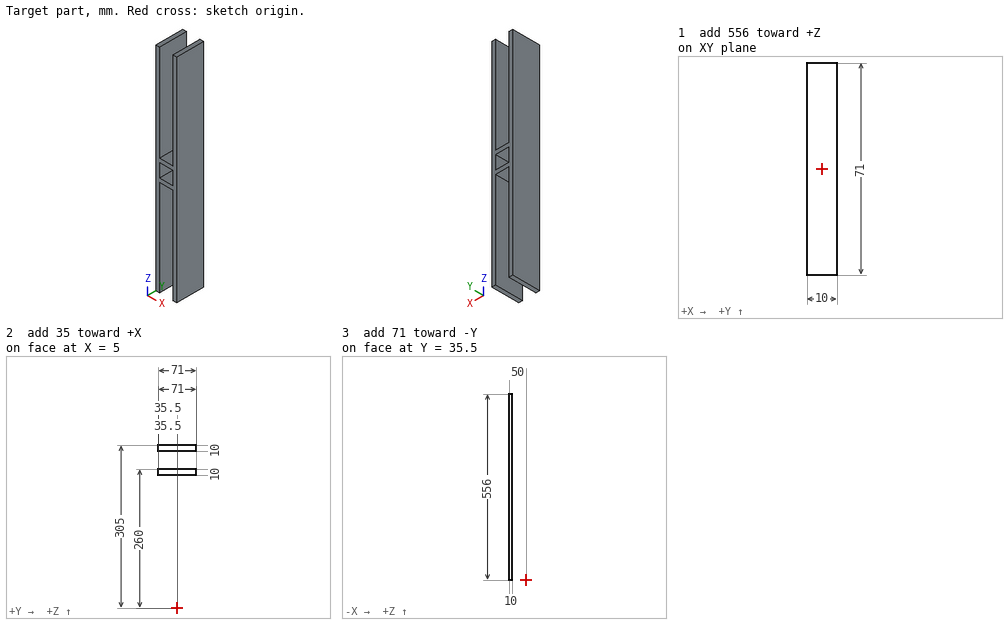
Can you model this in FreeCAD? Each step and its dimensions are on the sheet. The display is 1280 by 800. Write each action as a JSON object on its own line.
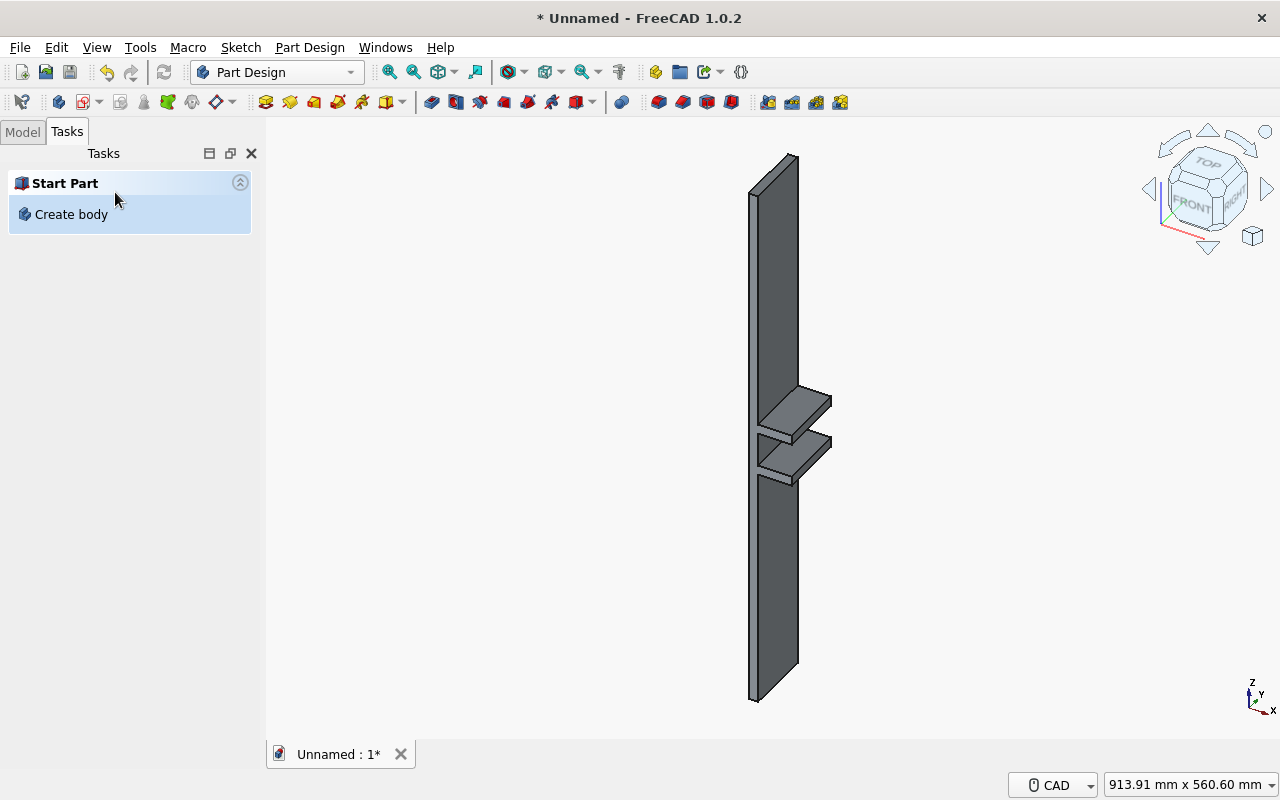
{"action": "key", "text": "4"}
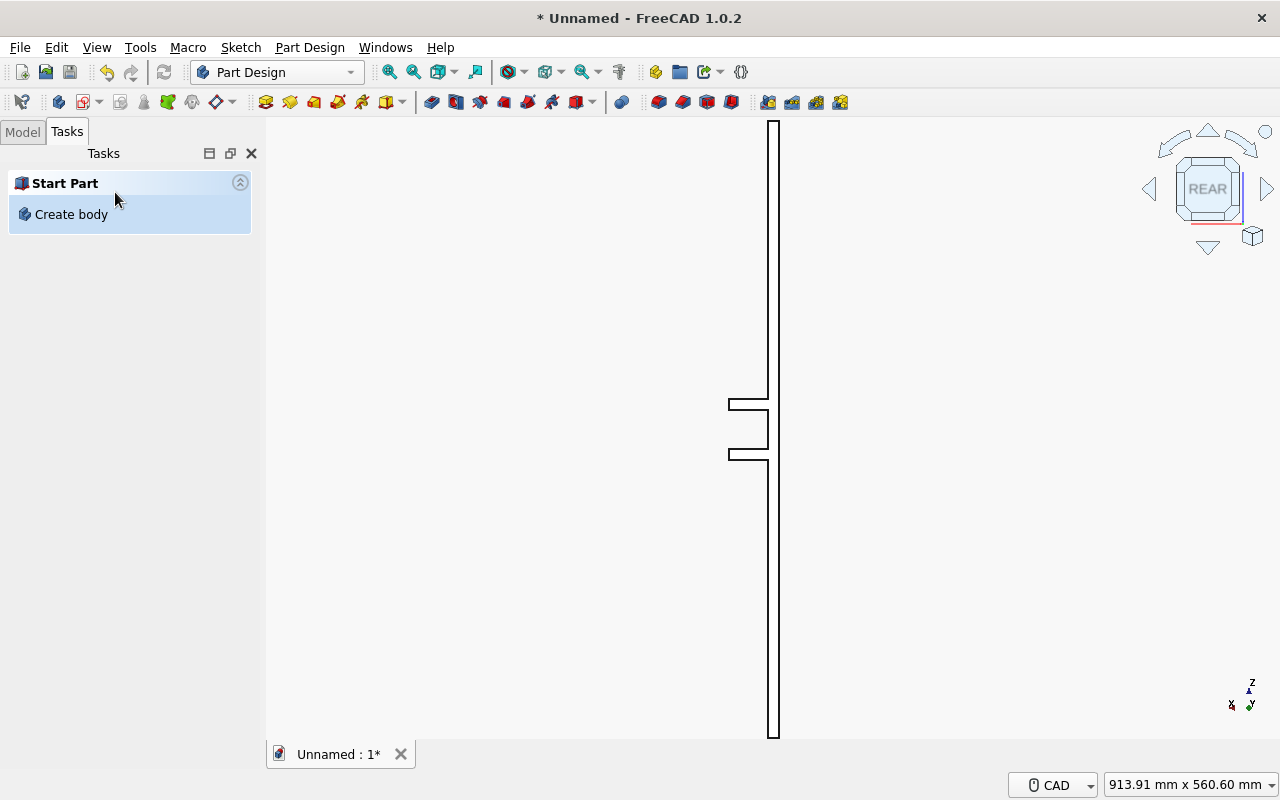
{"action": "scroll", "coordinate": [776, 164], "scroll_direction": "up", "scroll_amount": 7}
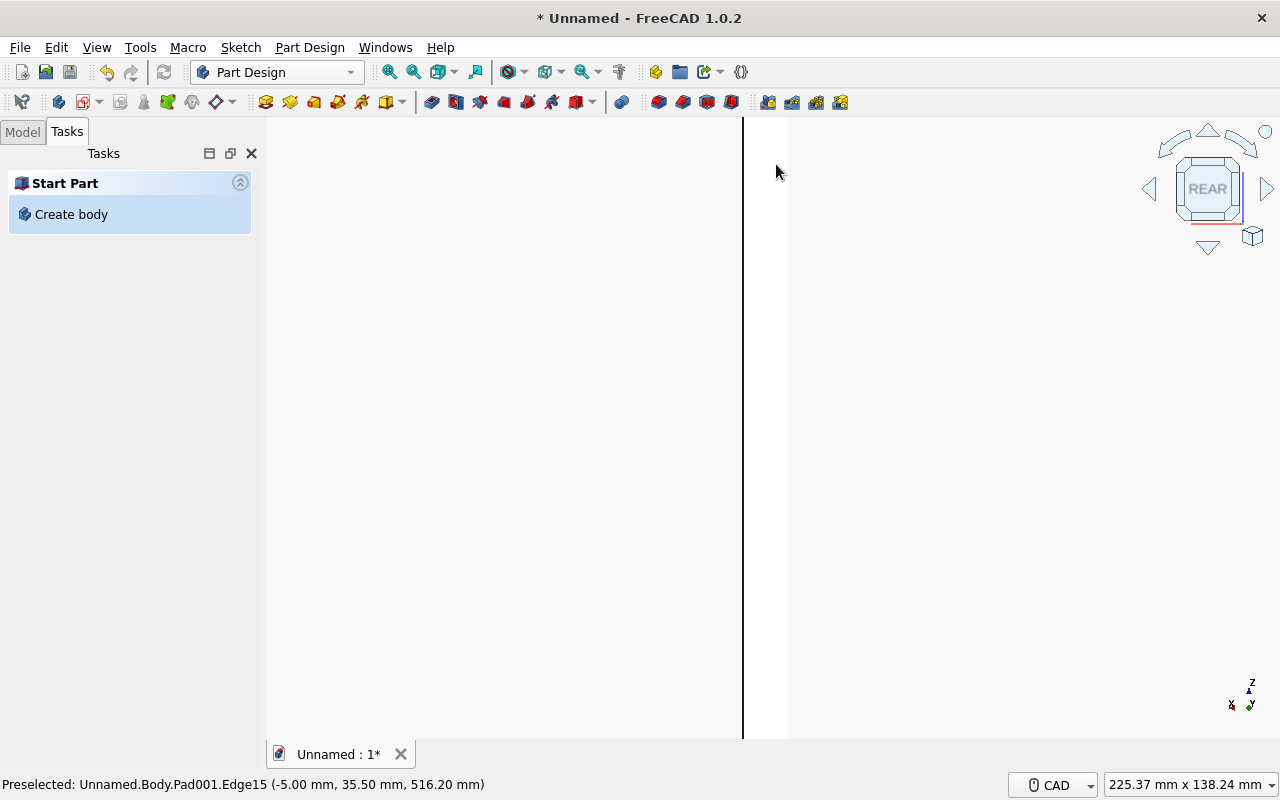
{"action": "left_click", "coordinate": [774, 166]}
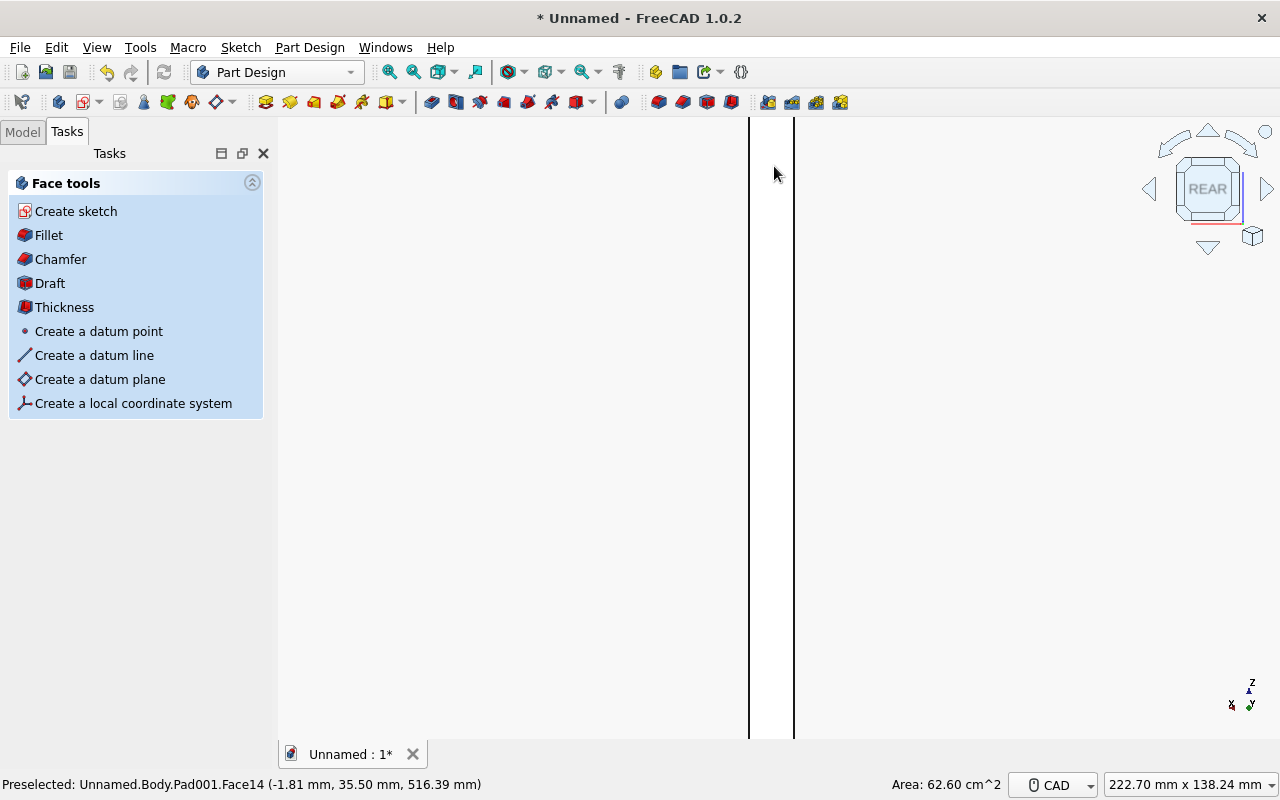
{"action": "left_click", "coordinate": [84, 102]}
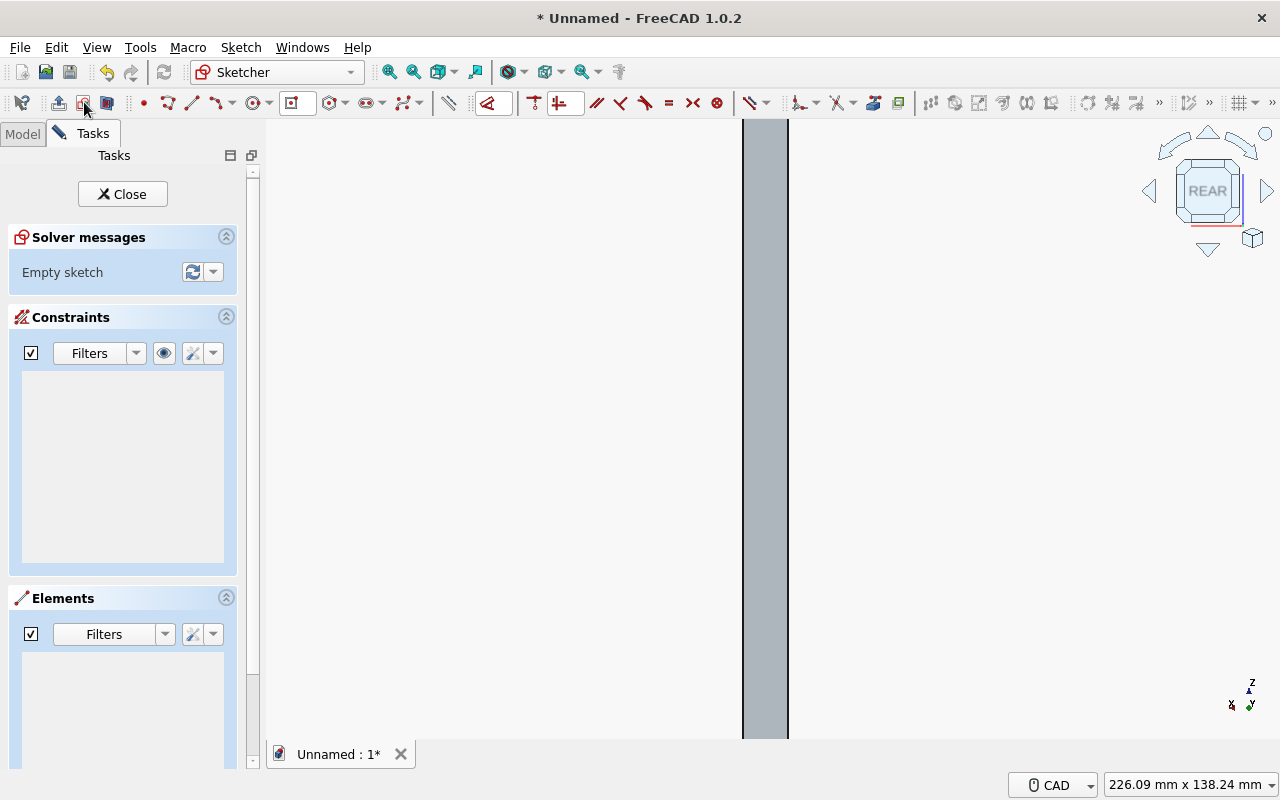
{"action": "scroll", "coordinate": [715, 269], "scroll_direction": "down", "scroll_amount": 9}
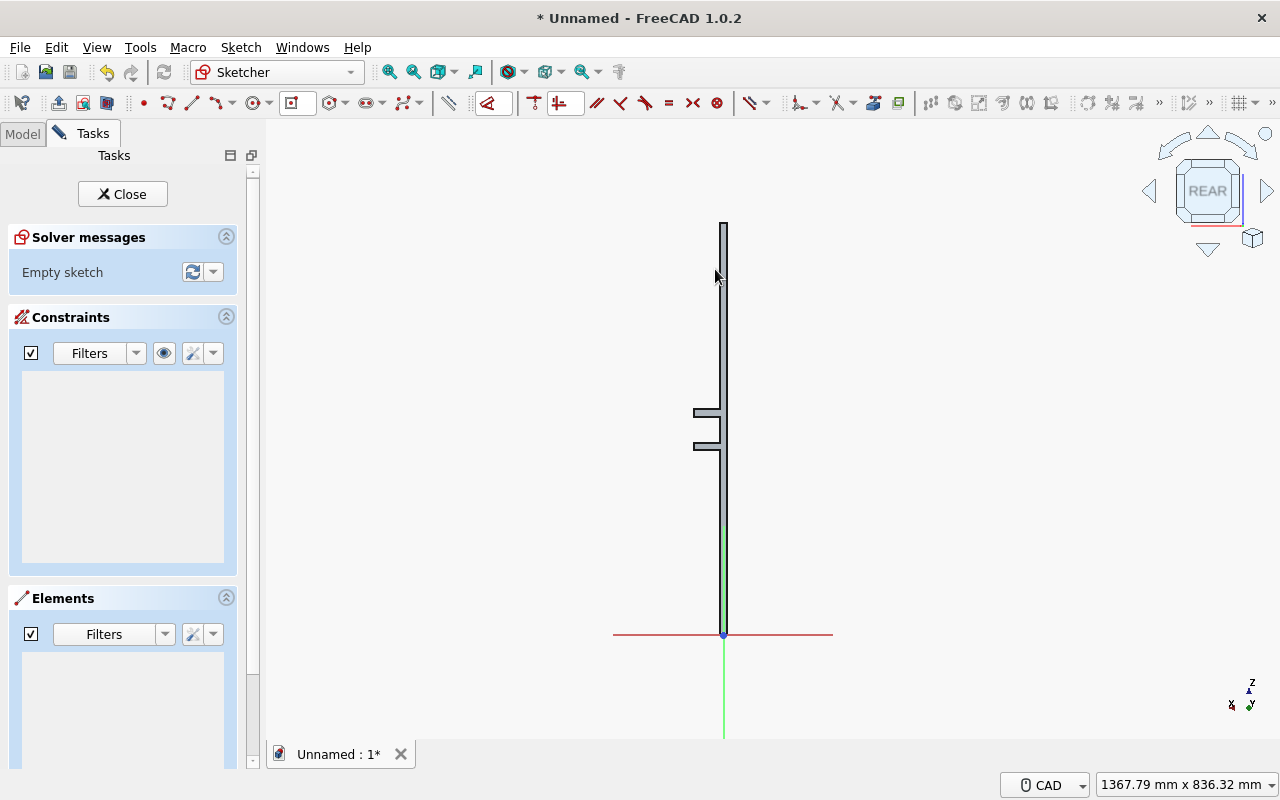
{"action": "key", "text": "g r"}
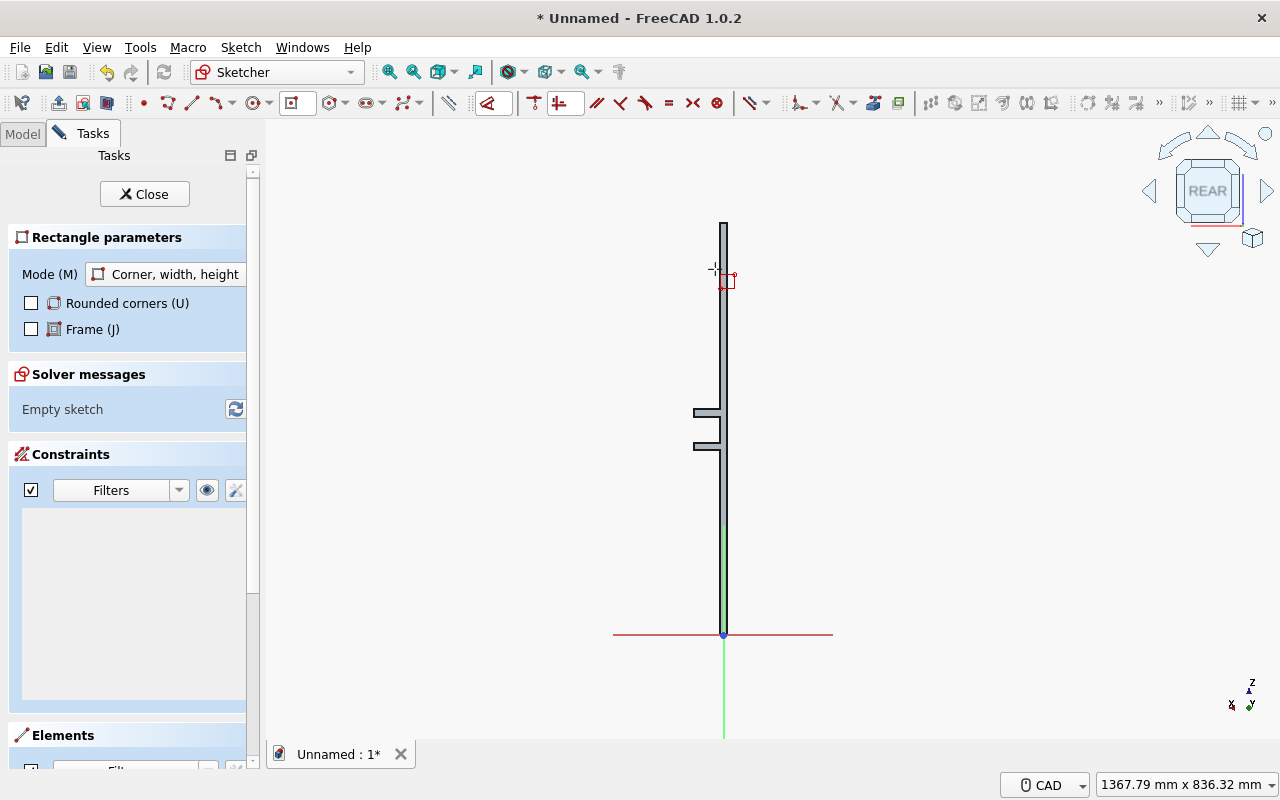
{"action": "scroll", "coordinate": [687, 223], "scroll_direction": "up", "scroll_amount": 4}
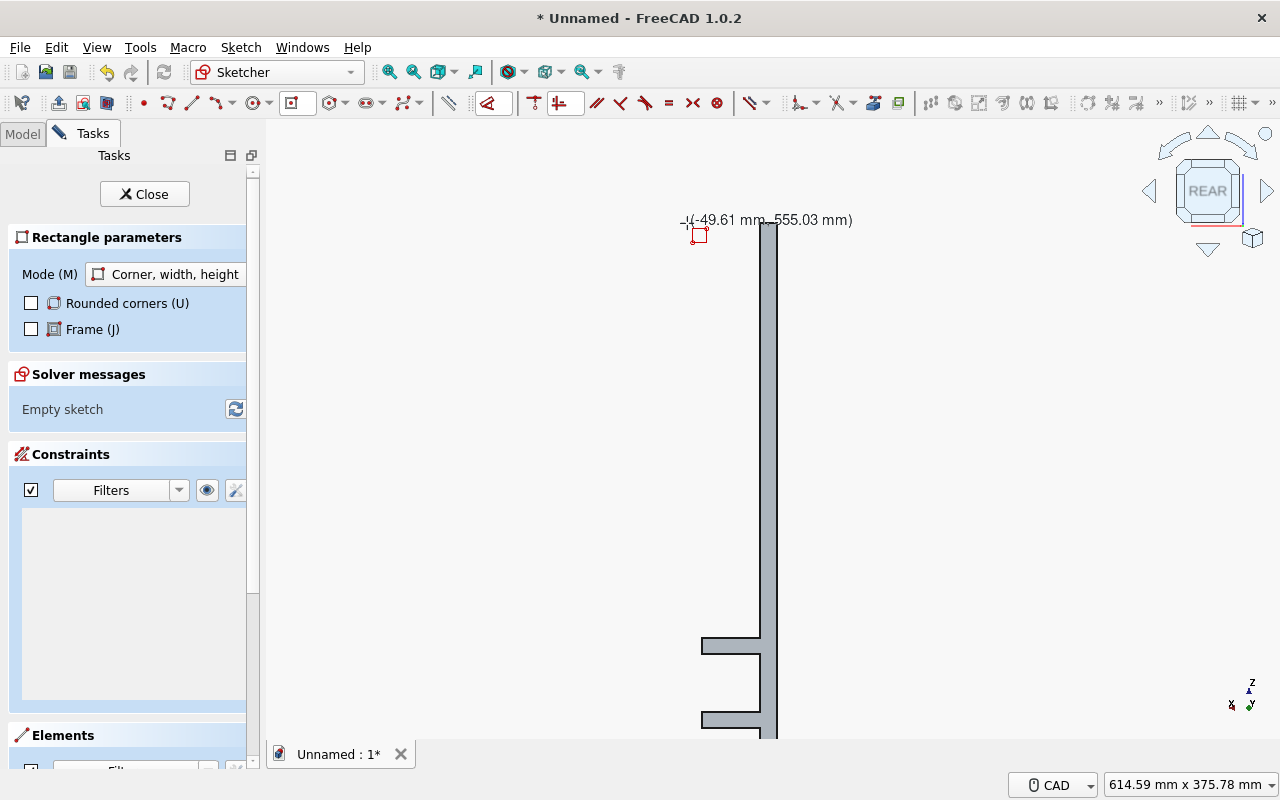
{"action": "left_click", "coordinate": [686, 223]}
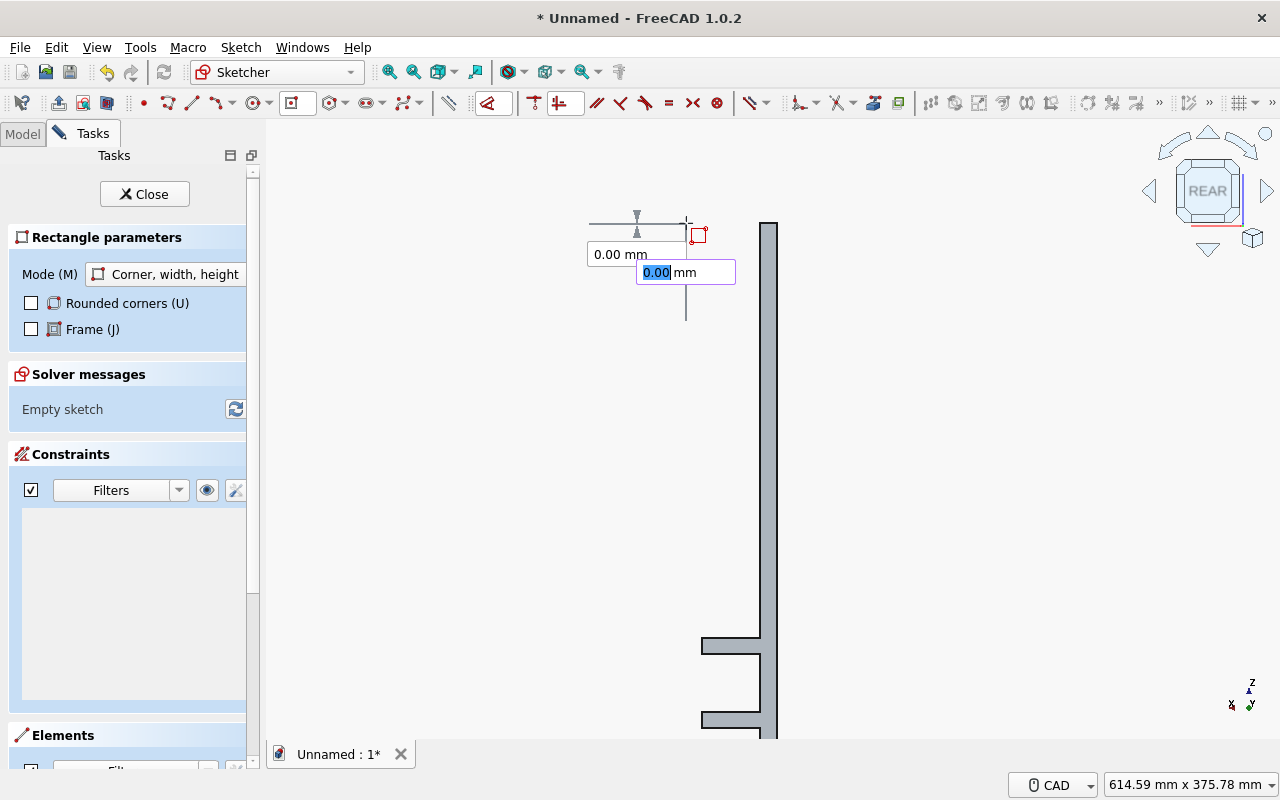
{"action": "scroll", "coordinate": [686, 222], "scroll_direction": "down", "scroll_amount": 4}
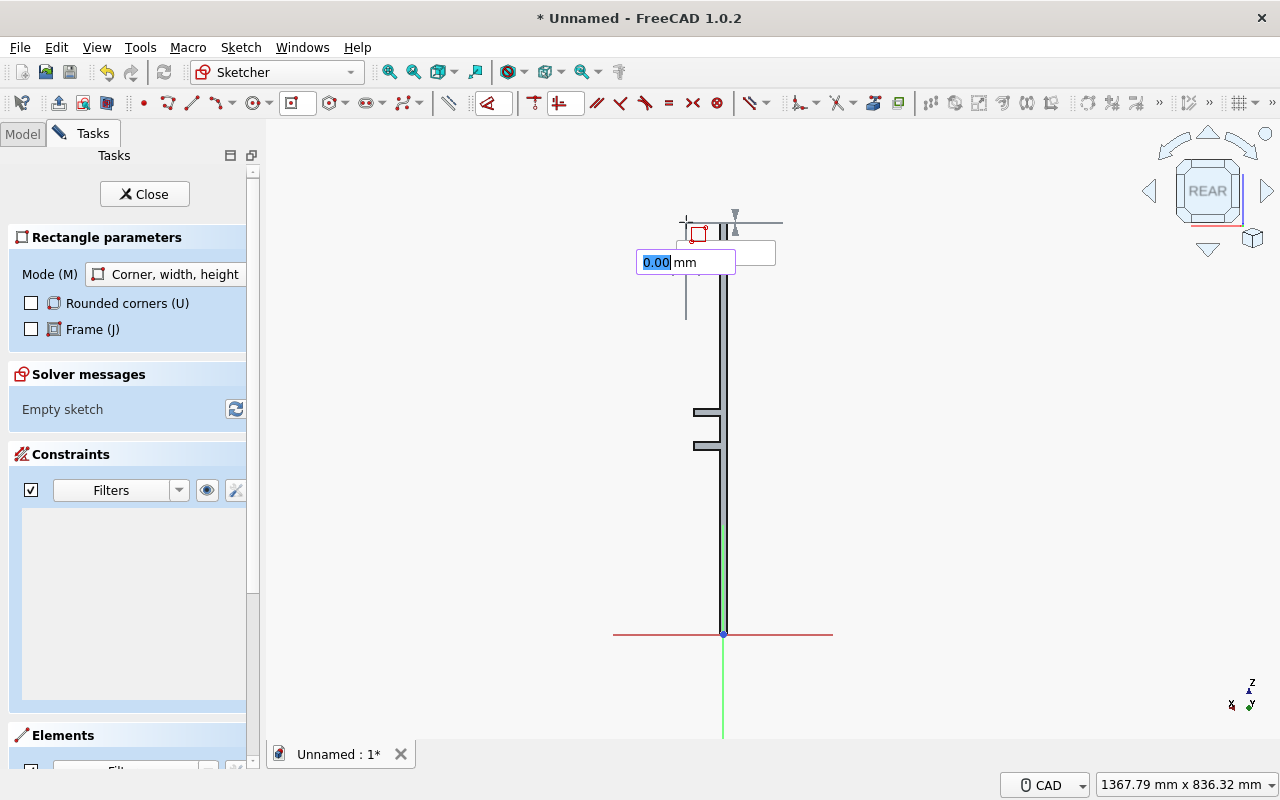
{"action": "left_click", "coordinate": [694, 635]}
{"action": "key", "text": "Escape"}